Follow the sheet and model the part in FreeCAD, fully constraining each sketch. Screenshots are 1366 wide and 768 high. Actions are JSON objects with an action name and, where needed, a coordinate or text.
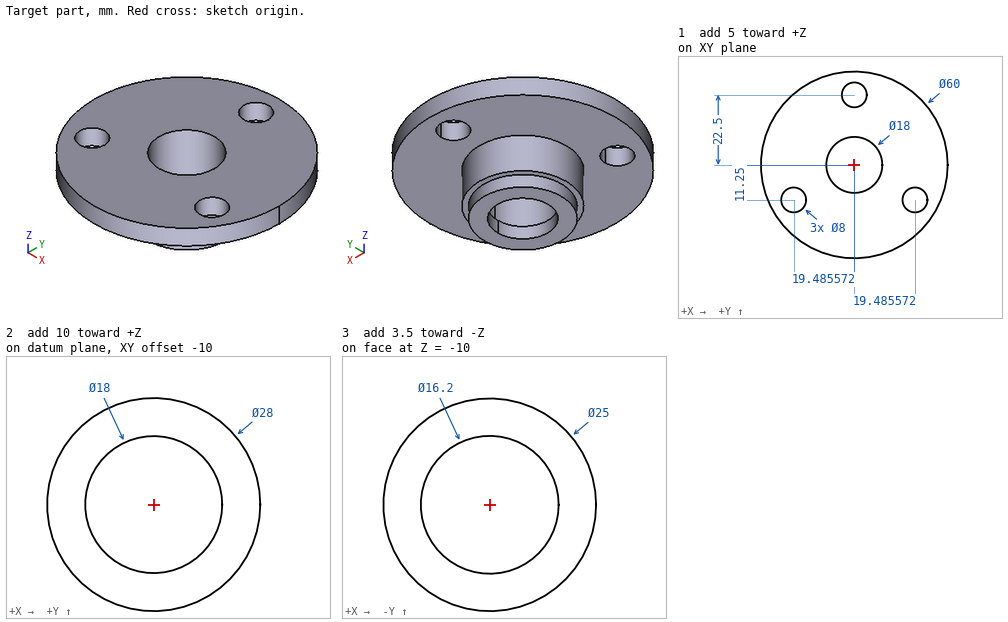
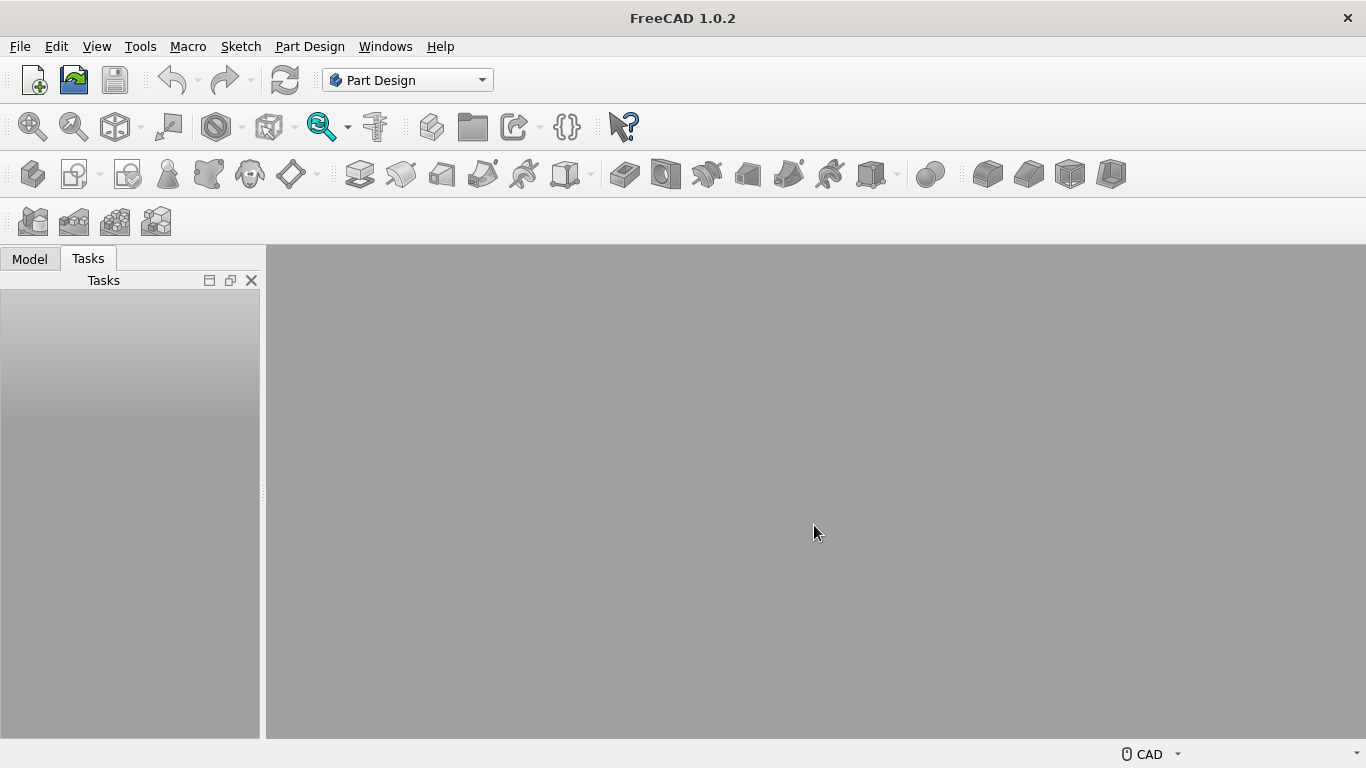
{"action": "left_click", "coordinate": [33, 80]}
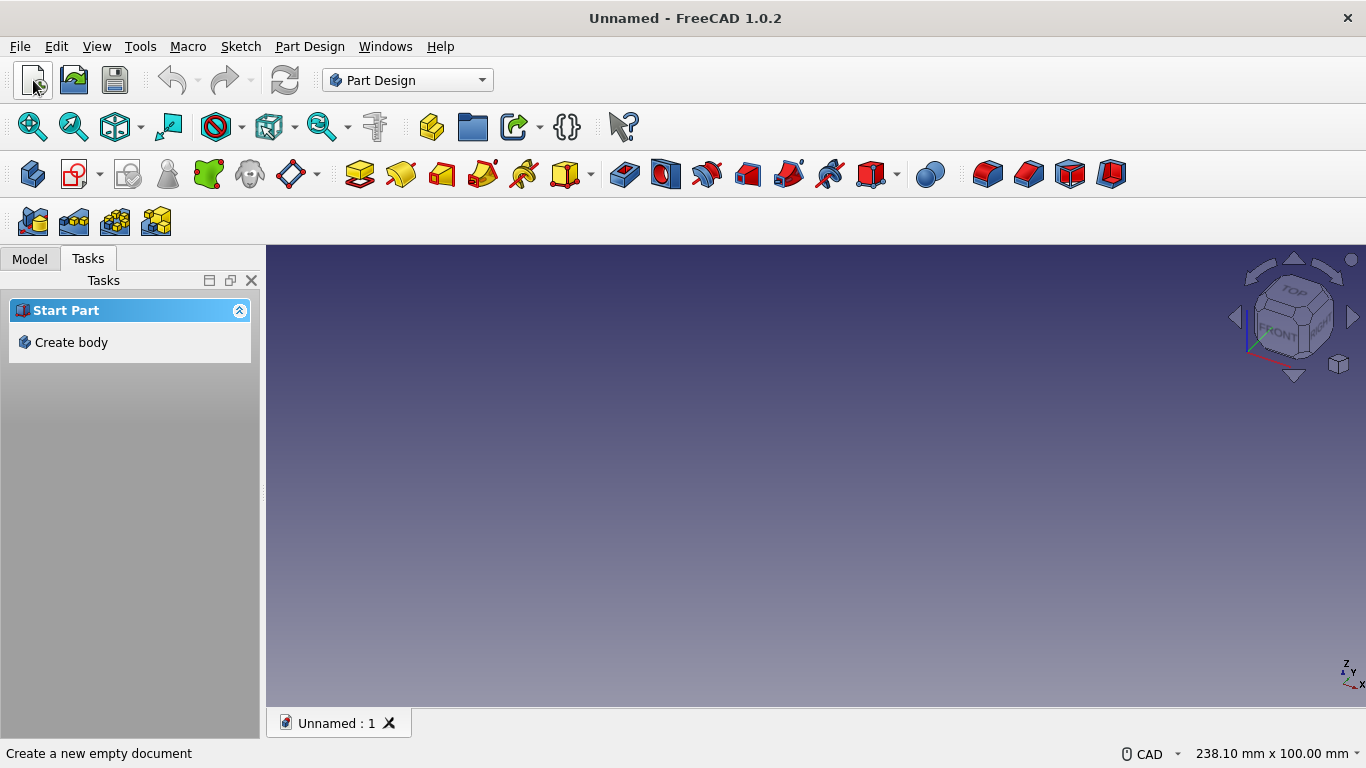
{"action": "left_click", "coordinate": [74, 174]}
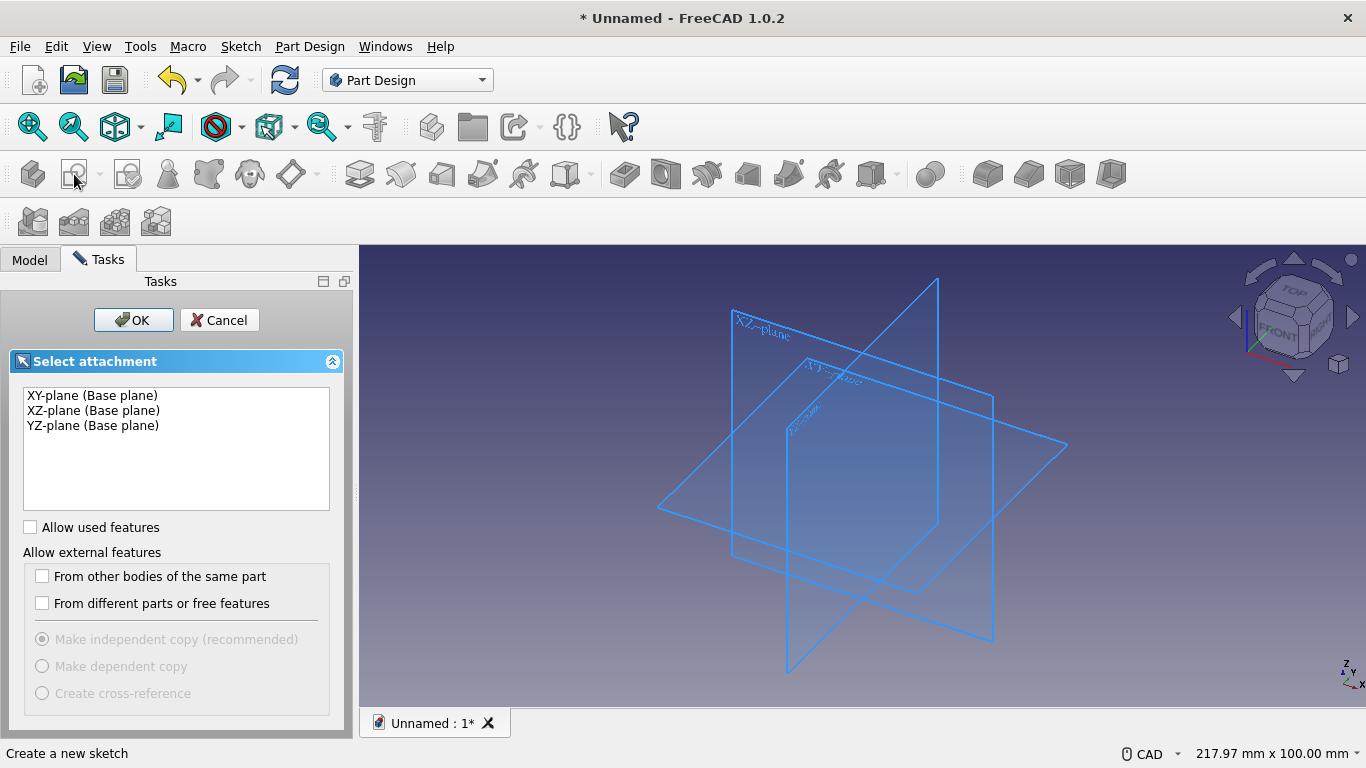
{"action": "left_click", "coordinate": [84, 396]}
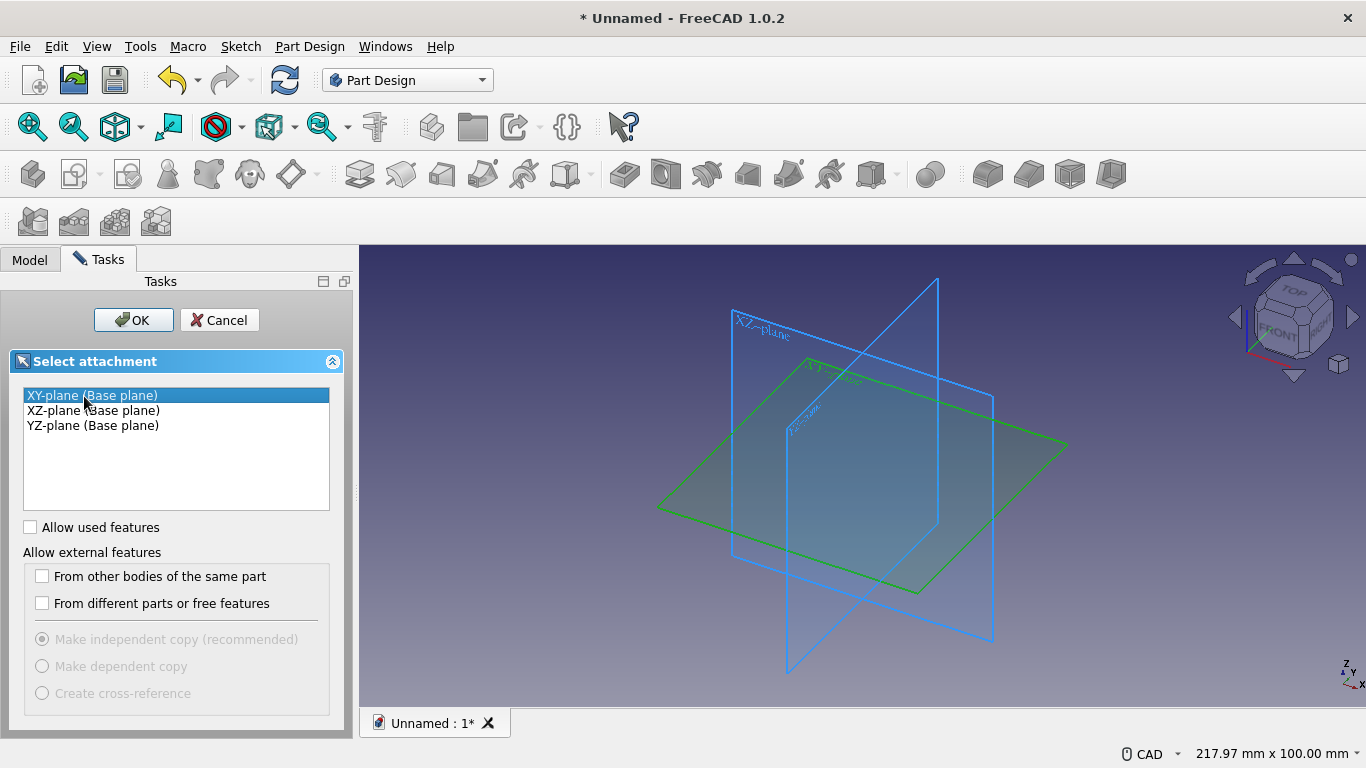
{"action": "left_click", "coordinate": [134, 320]}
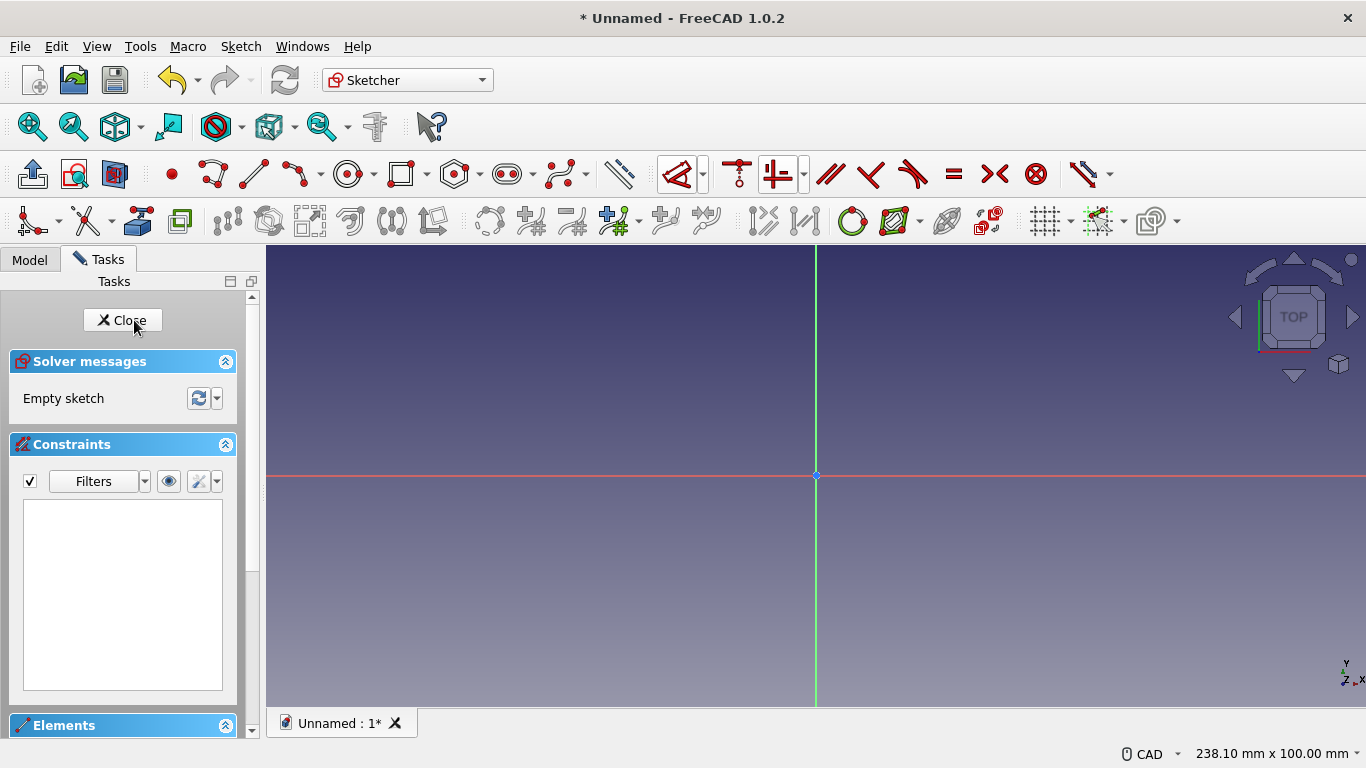
{"action": "left_click", "coordinate": [348, 174]}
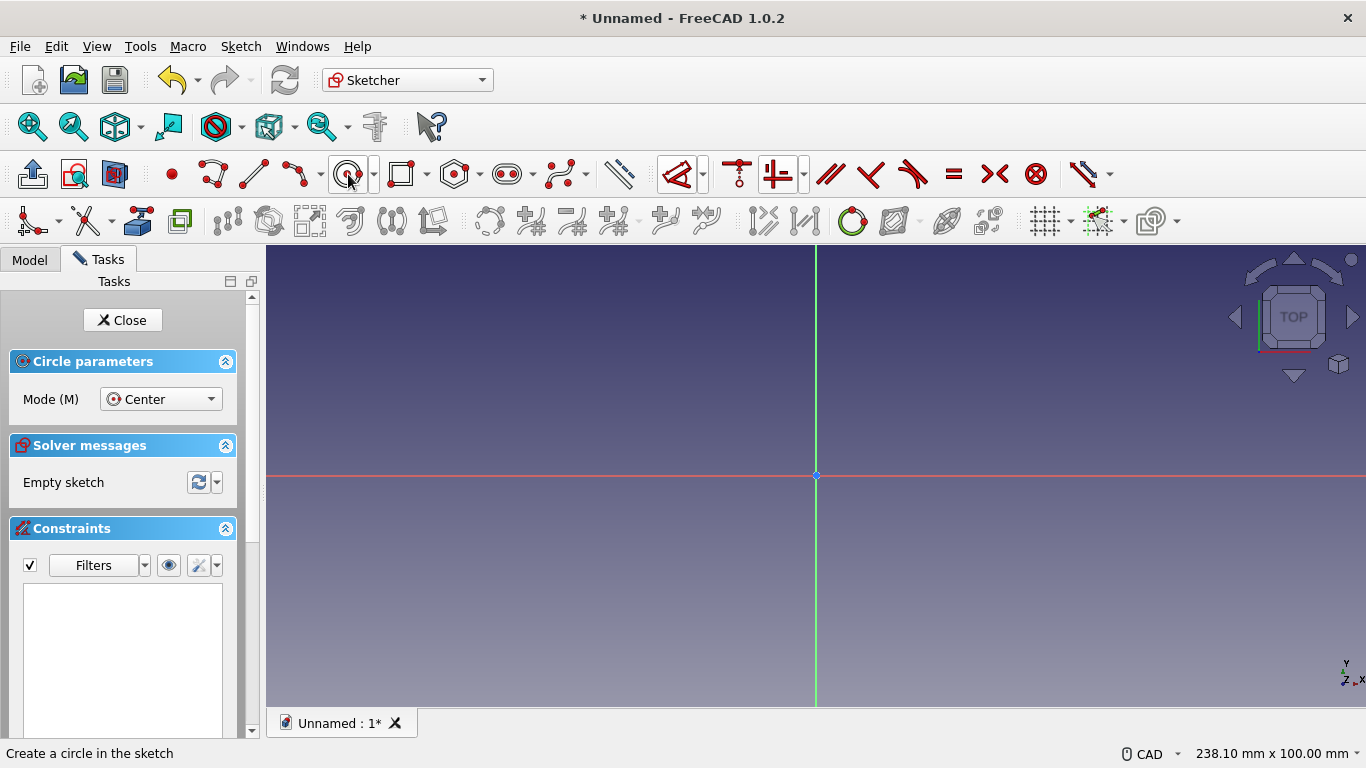
{"action": "left_click", "coordinate": [816, 476]}
{"action": "mouse_move", "coordinate": [914, 378]}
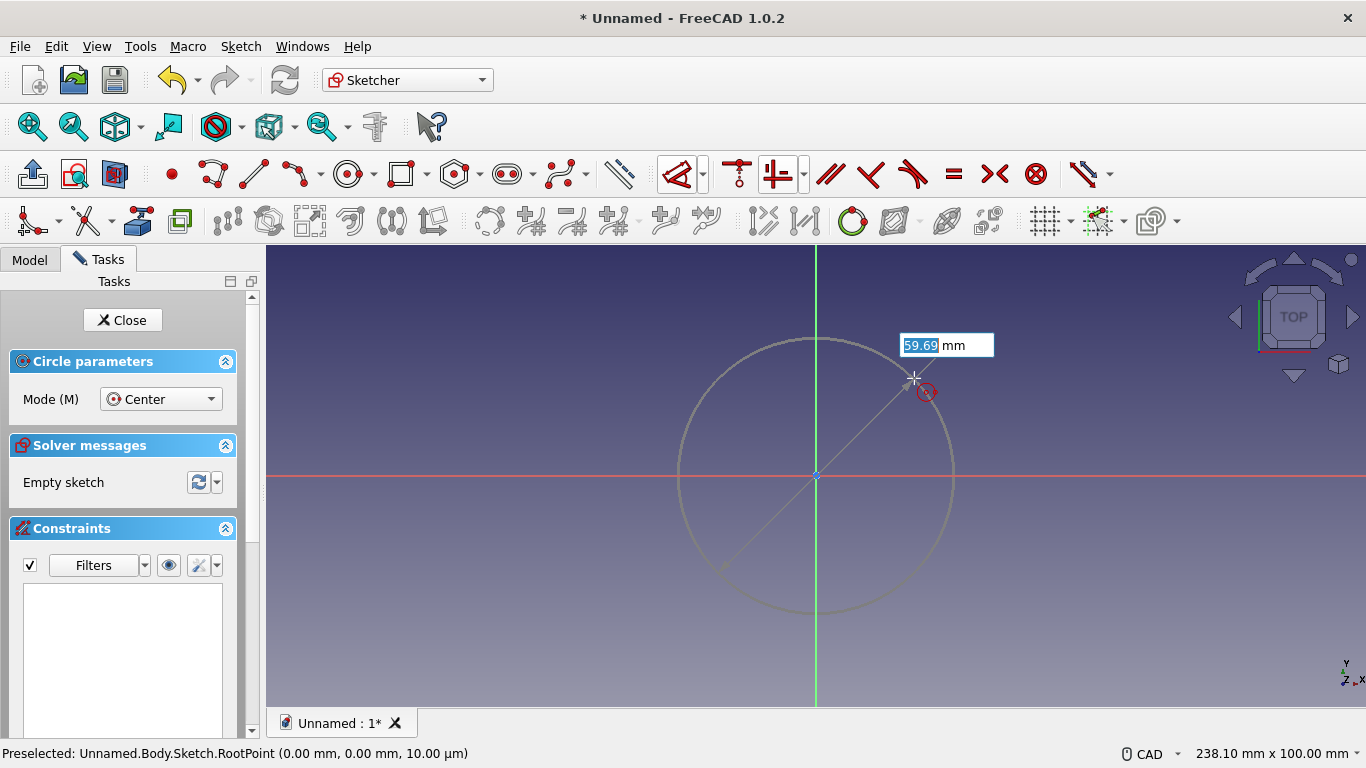
{"action": "type", "text": "60"}
{"action": "key", "text": "Return"}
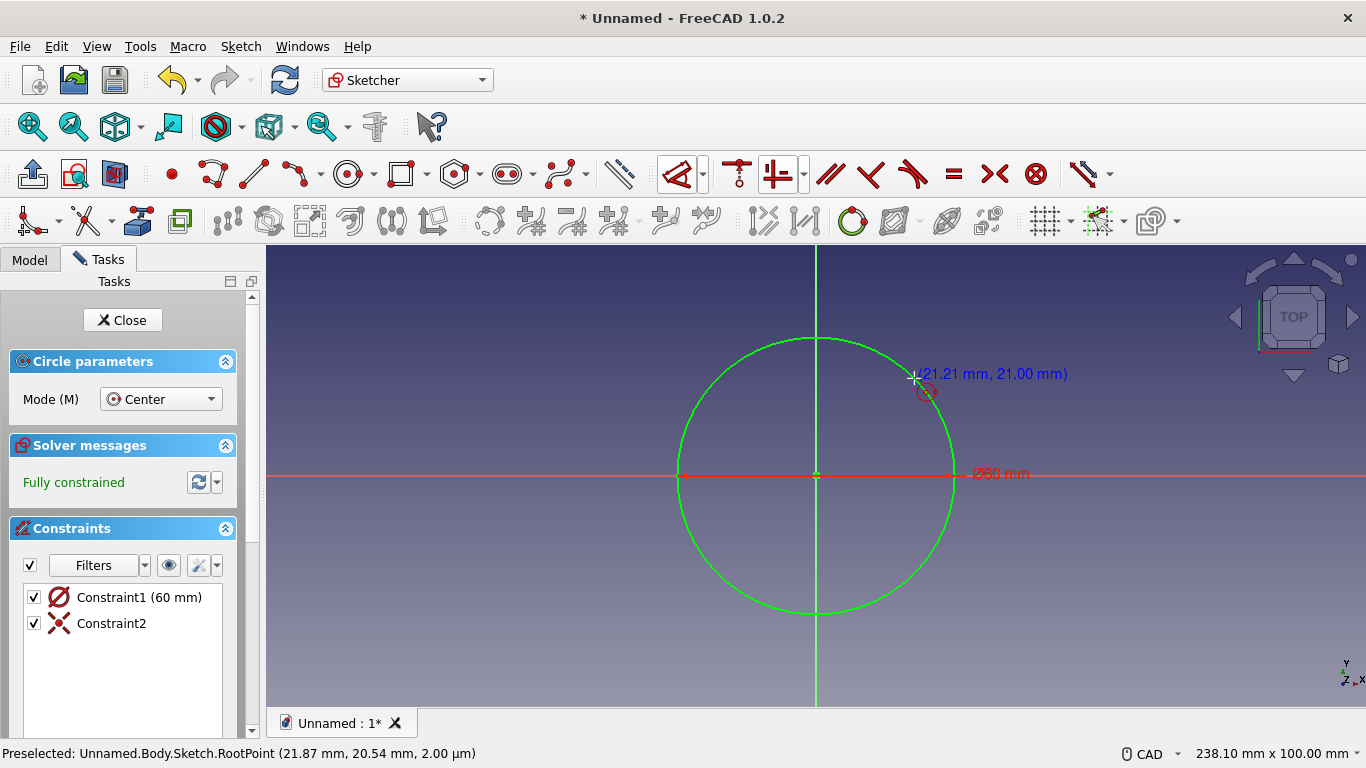
{"action": "scroll", "coordinate": [726, 528], "scroll_direction": "up", "scroll_amount": 2}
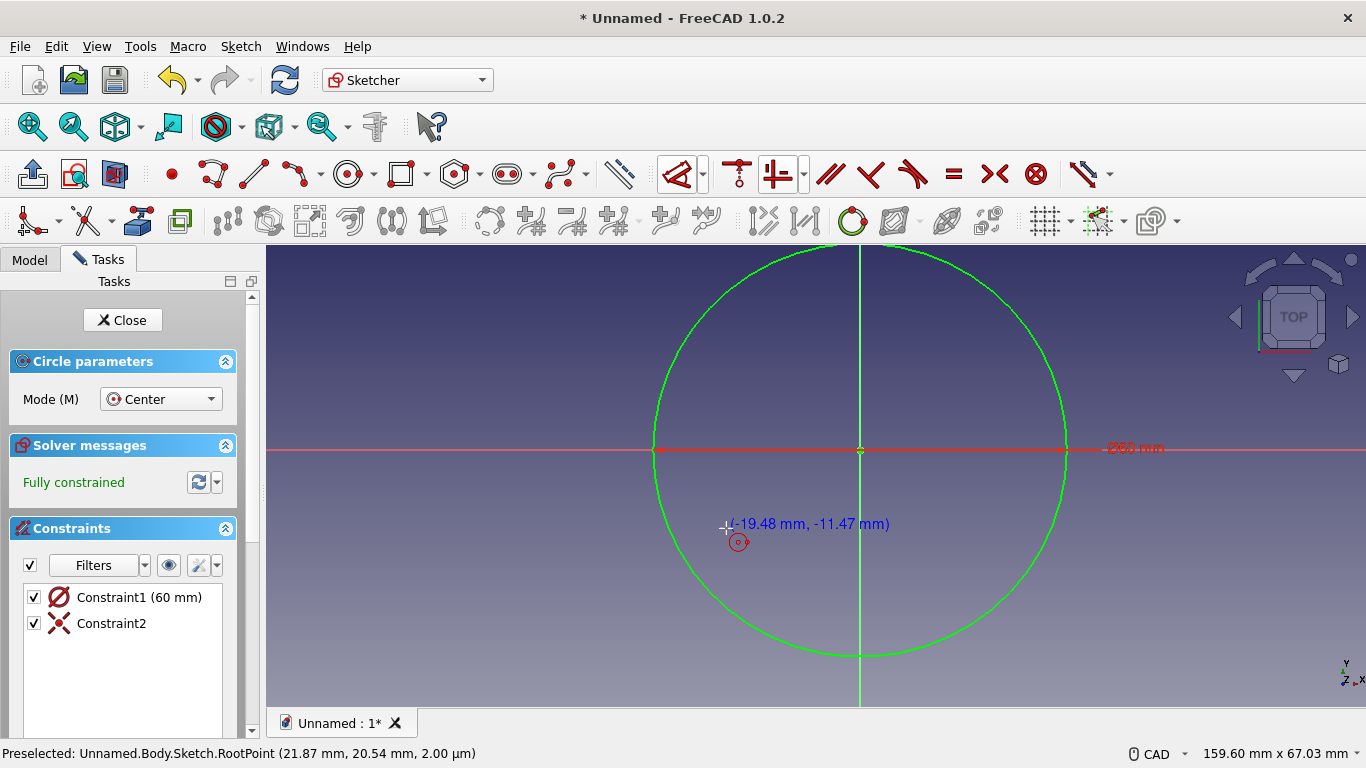
{"action": "left_click", "coordinate": [726, 528]}
{"action": "mouse_move", "coordinate": [745, 508]}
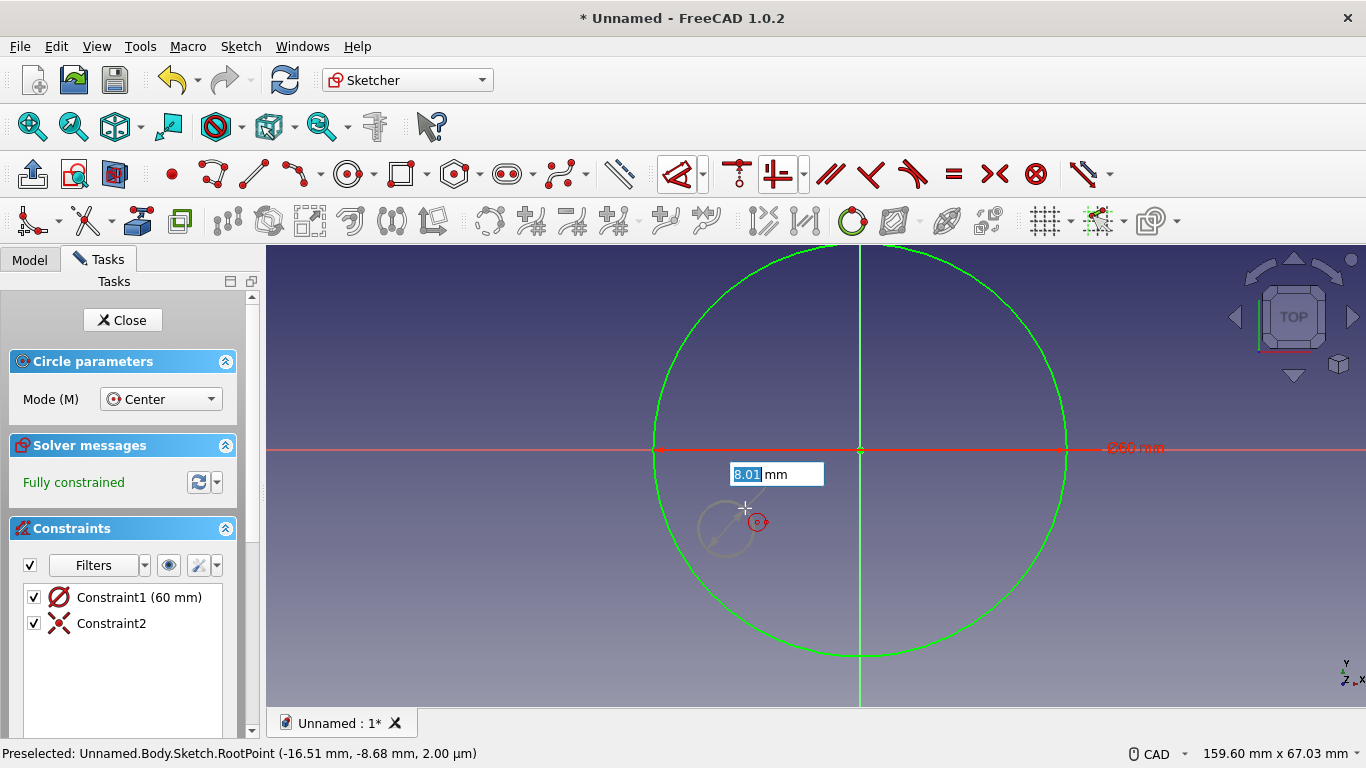
{"action": "type", "text": "8"}
{"action": "key", "text": "Return"}